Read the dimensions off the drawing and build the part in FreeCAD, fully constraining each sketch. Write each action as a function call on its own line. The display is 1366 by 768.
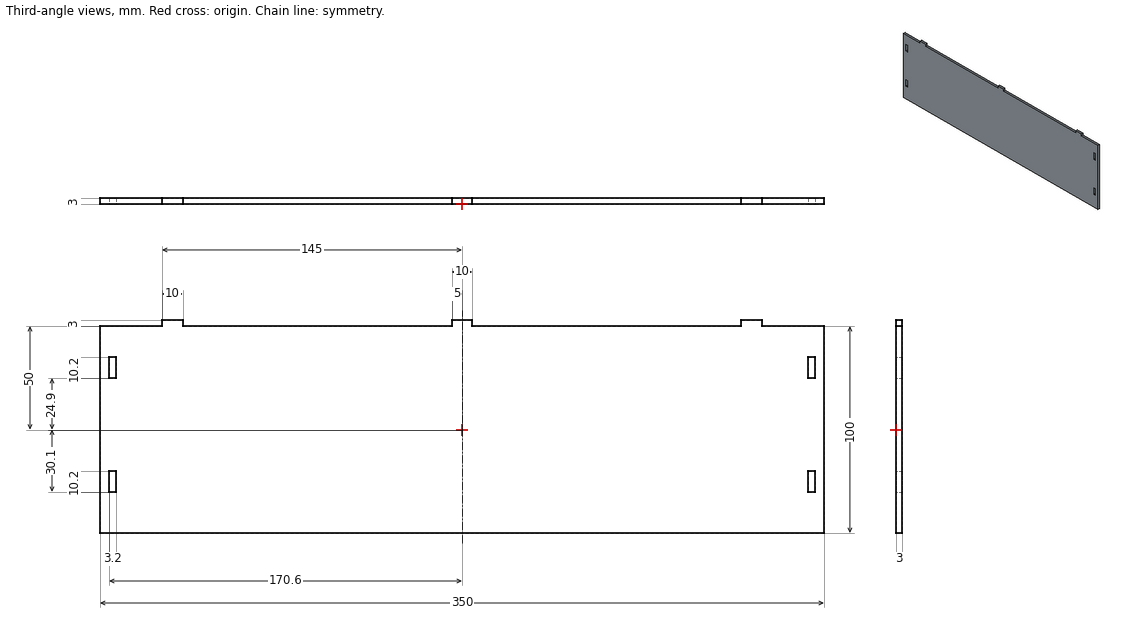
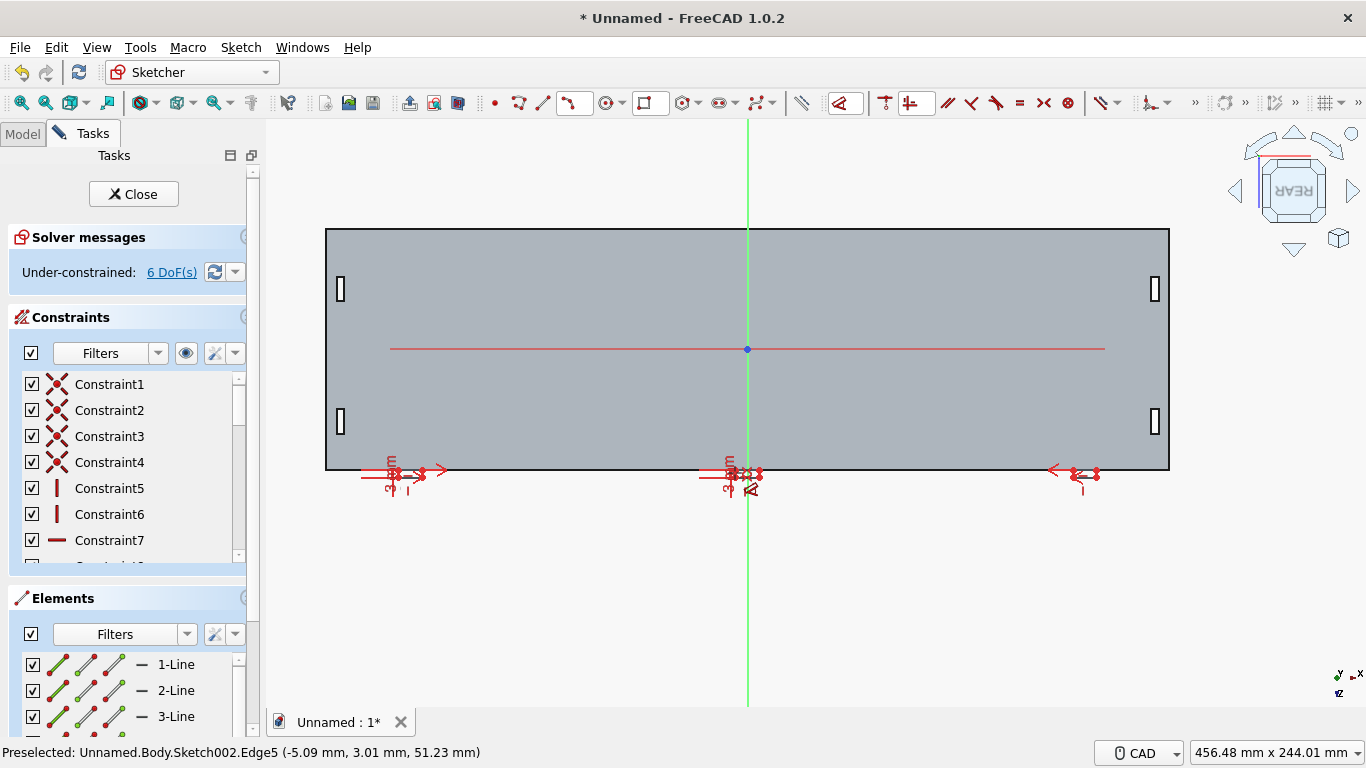
scroll(405, 478, up, 4)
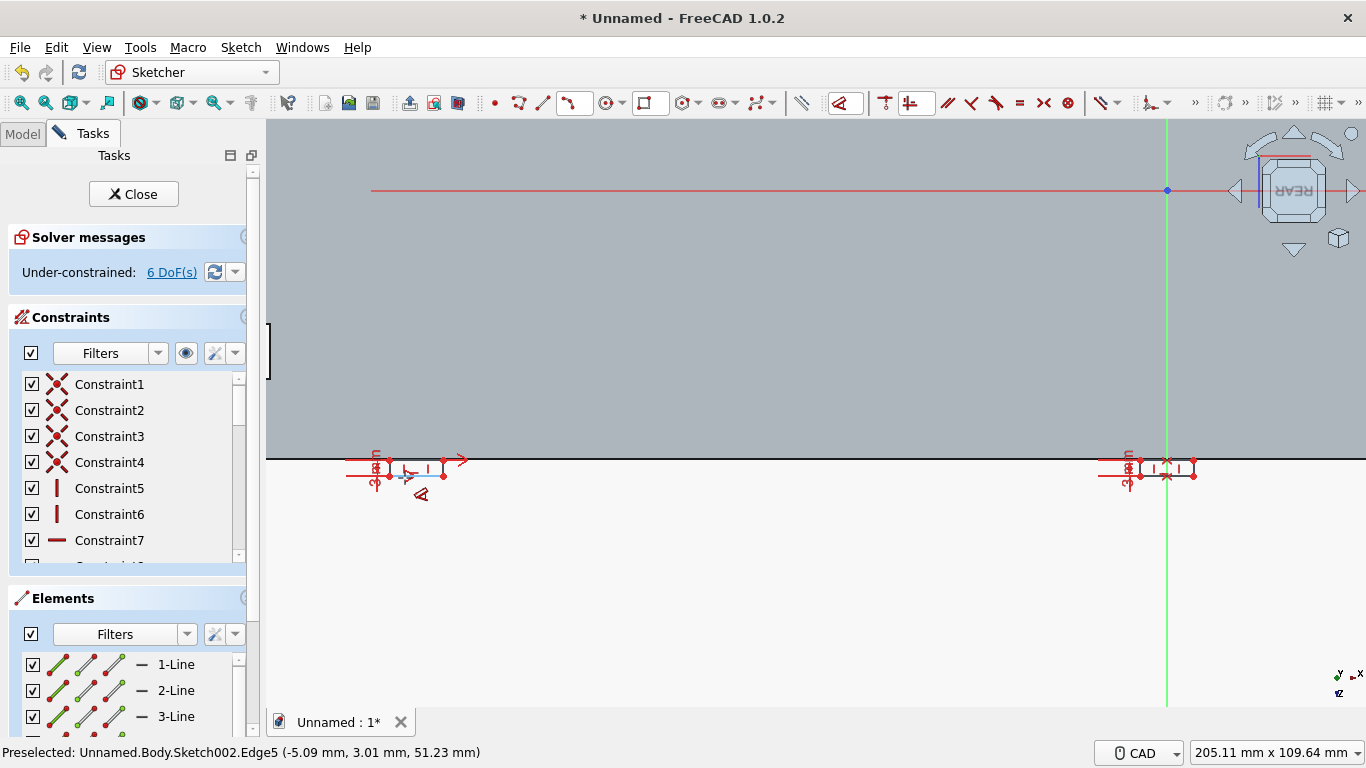
click(406, 476)
click(417, 510)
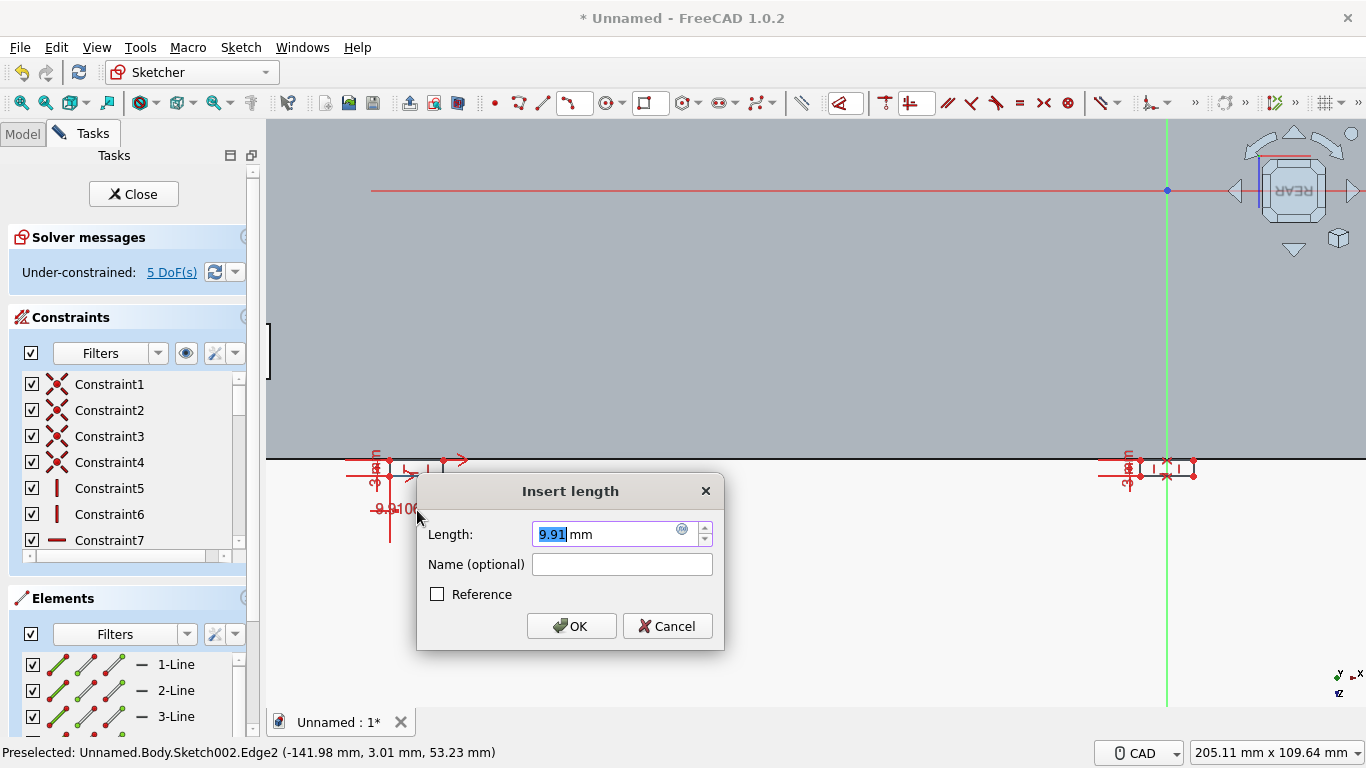
text(10)
key(Return)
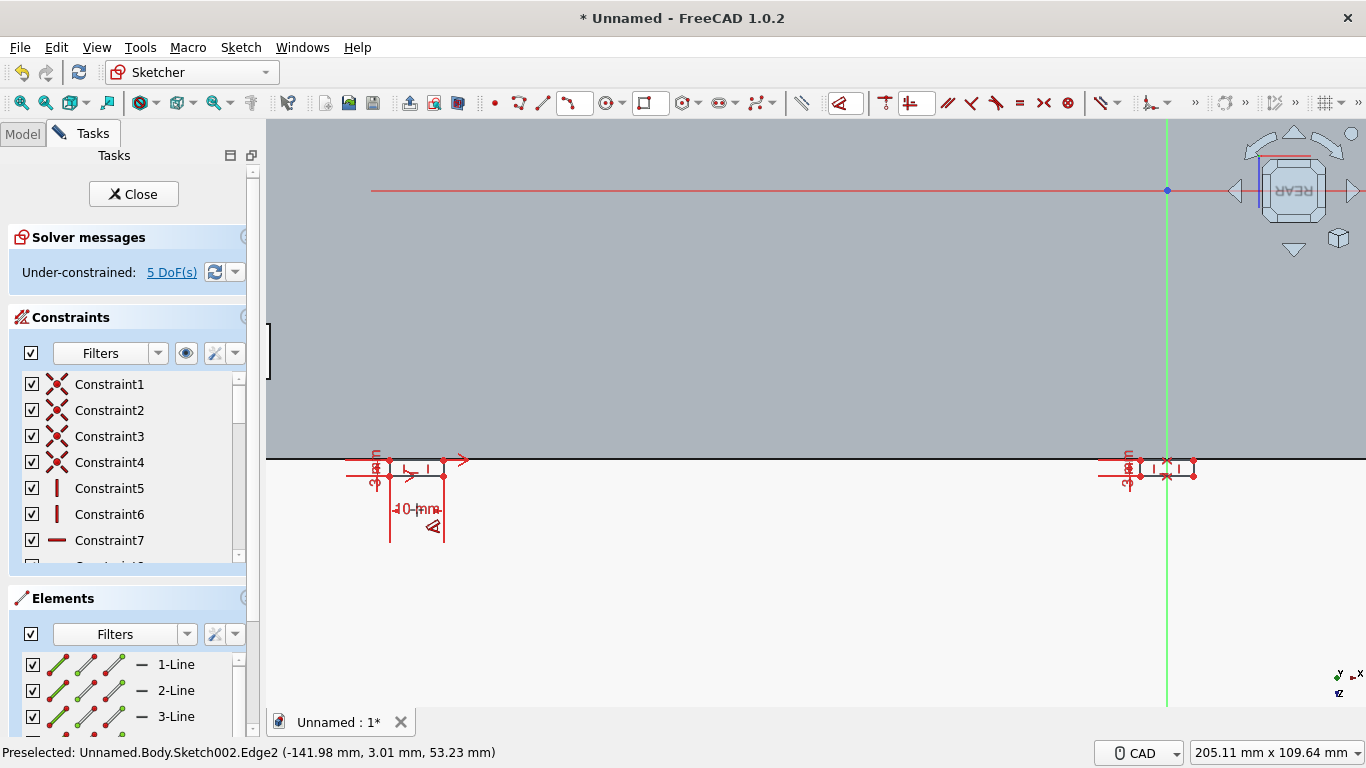
scroll(1156, 476, up, 2)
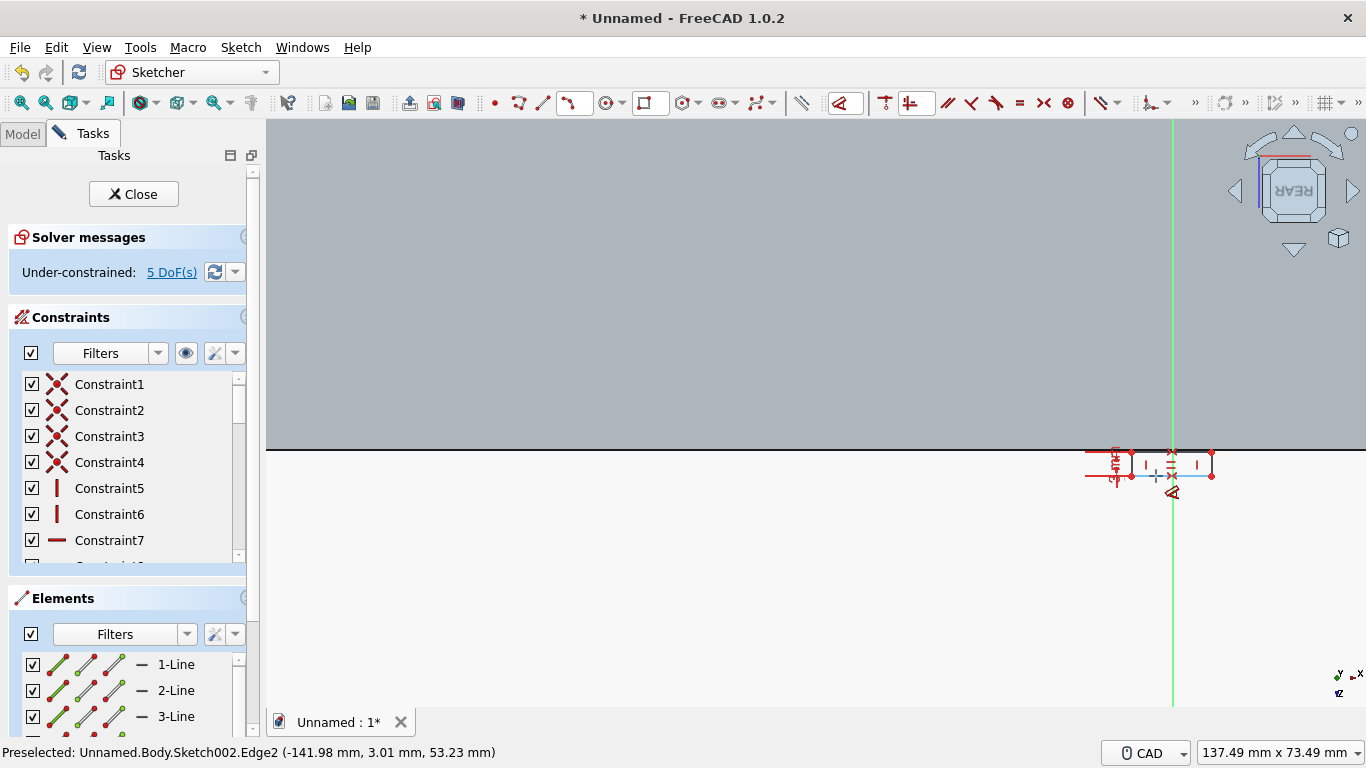
click(1156, 476)
click(1151, 510)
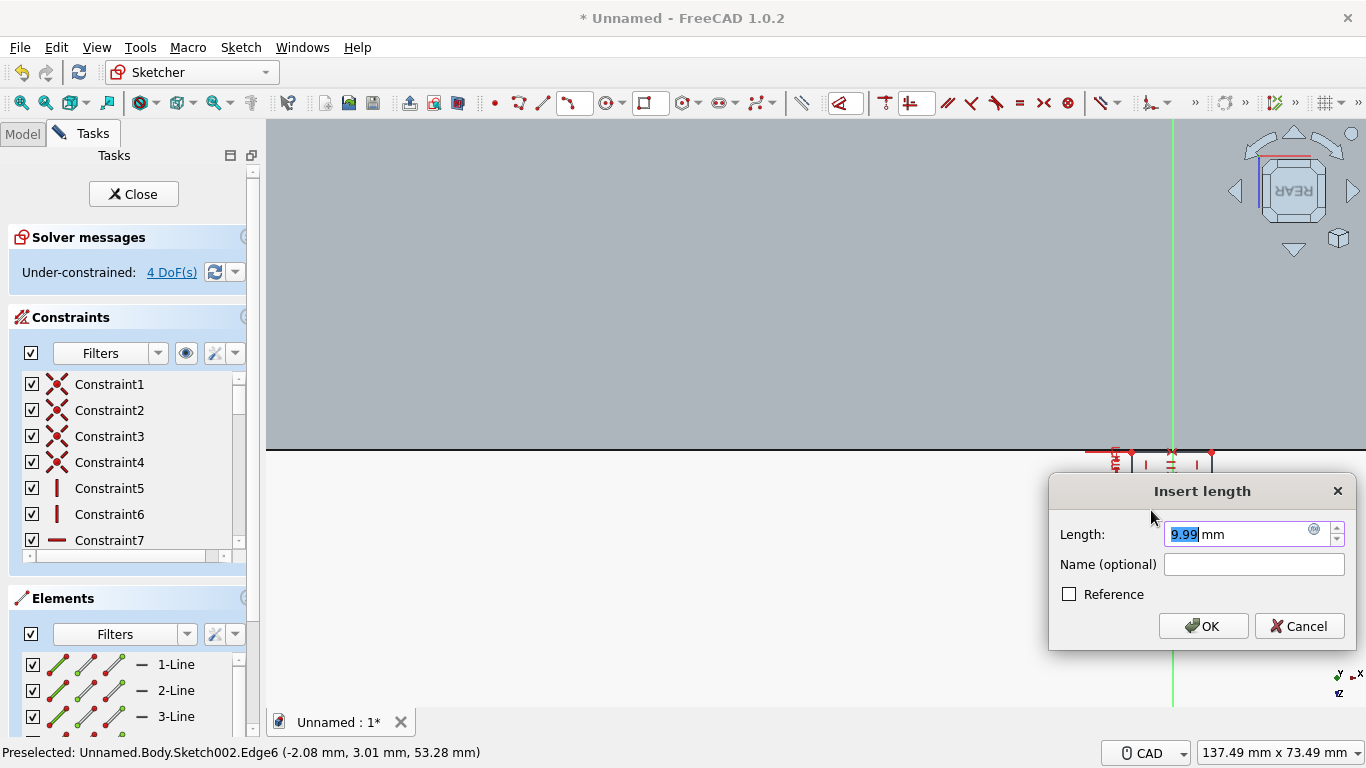
text(10)
key(Return)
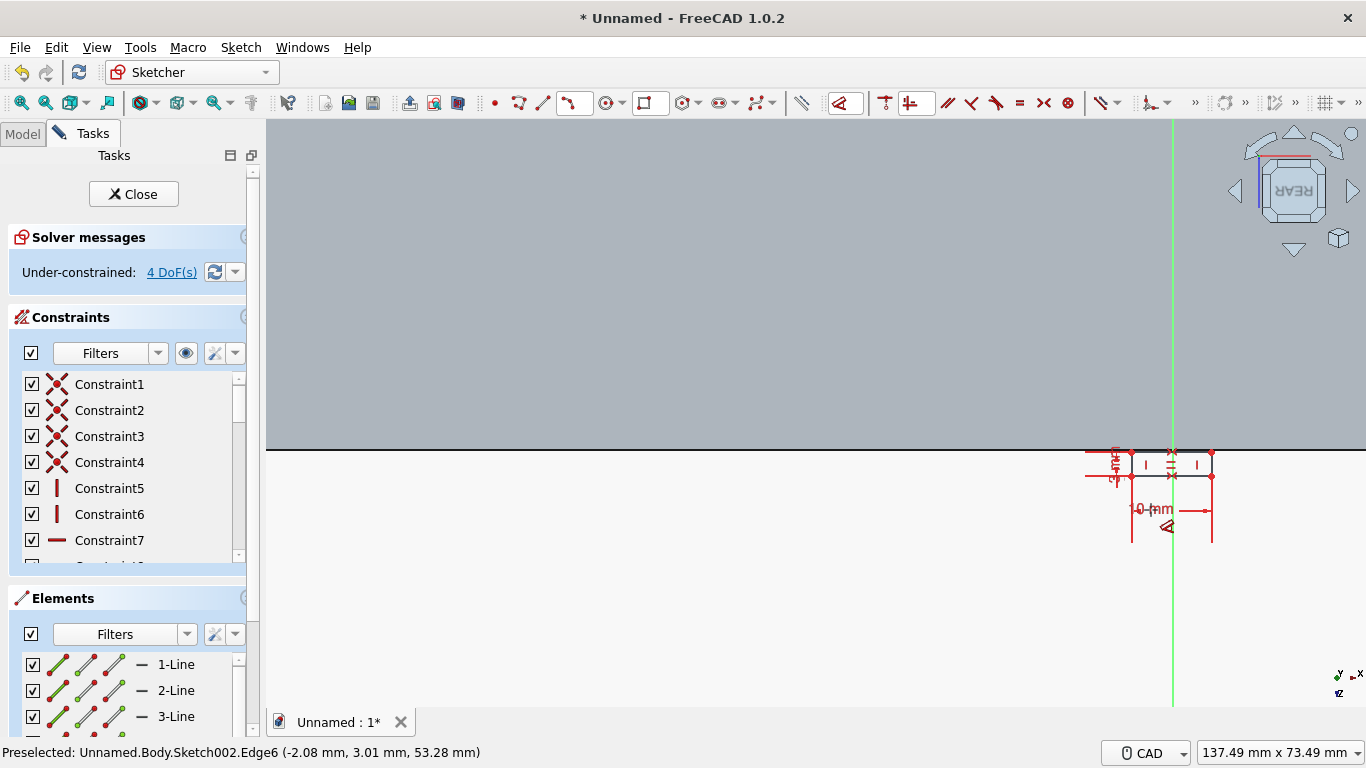
click(1132, 452)
click(1152, 534)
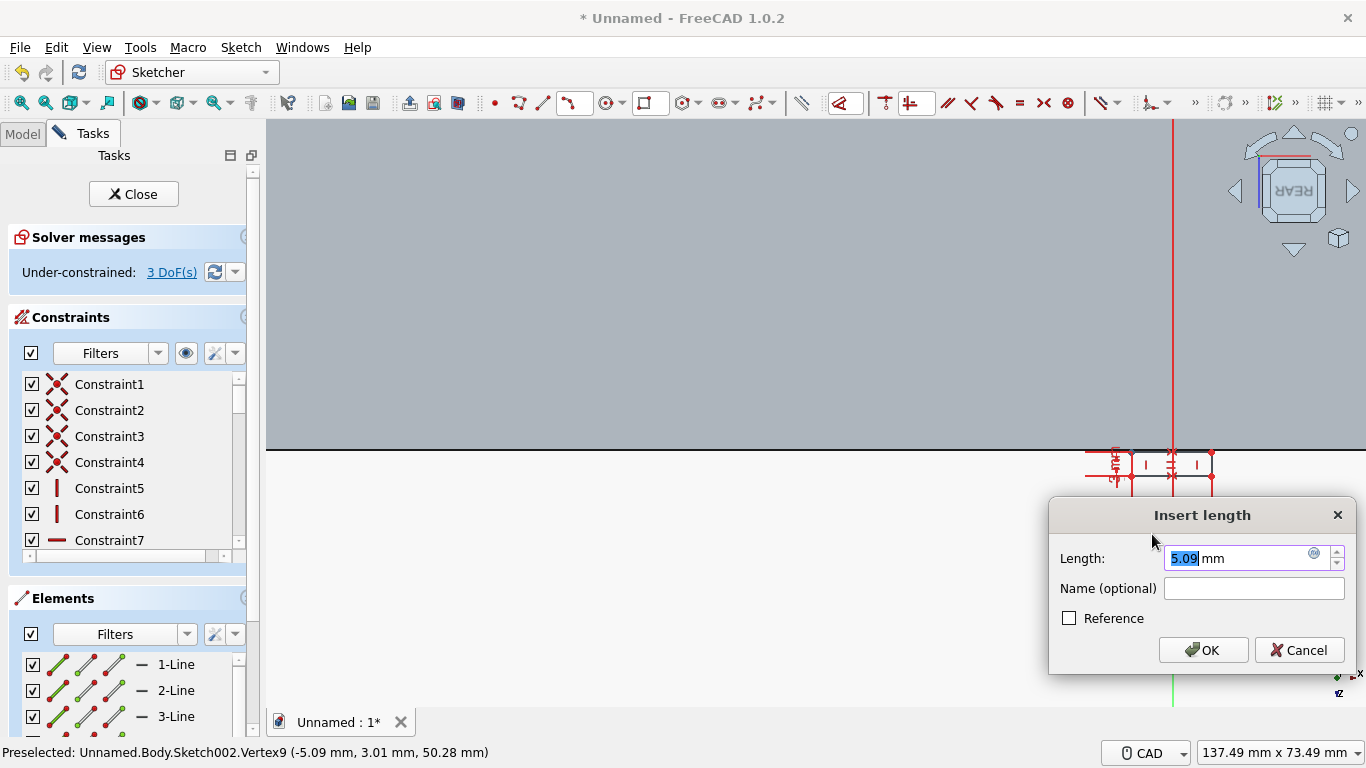
text(5)
key(Return)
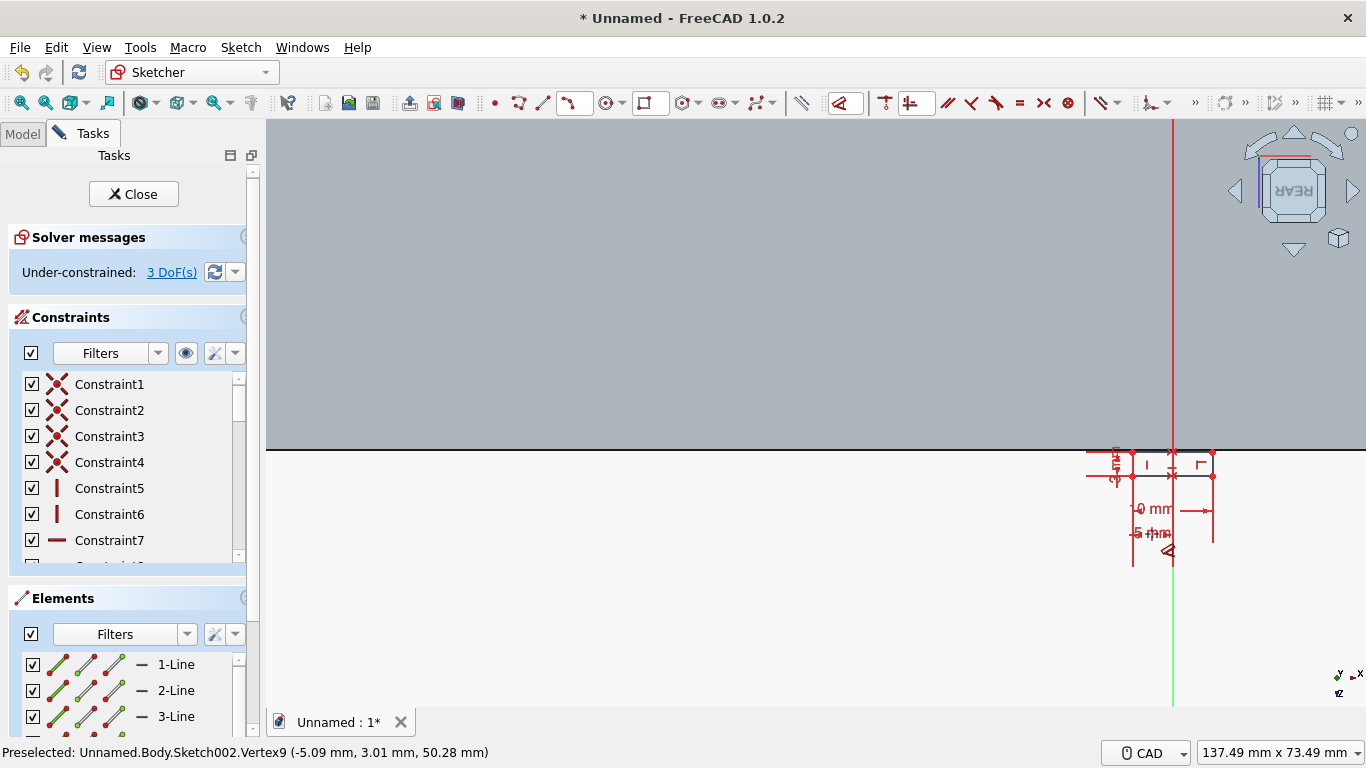
scroll(564, 478, down, 6)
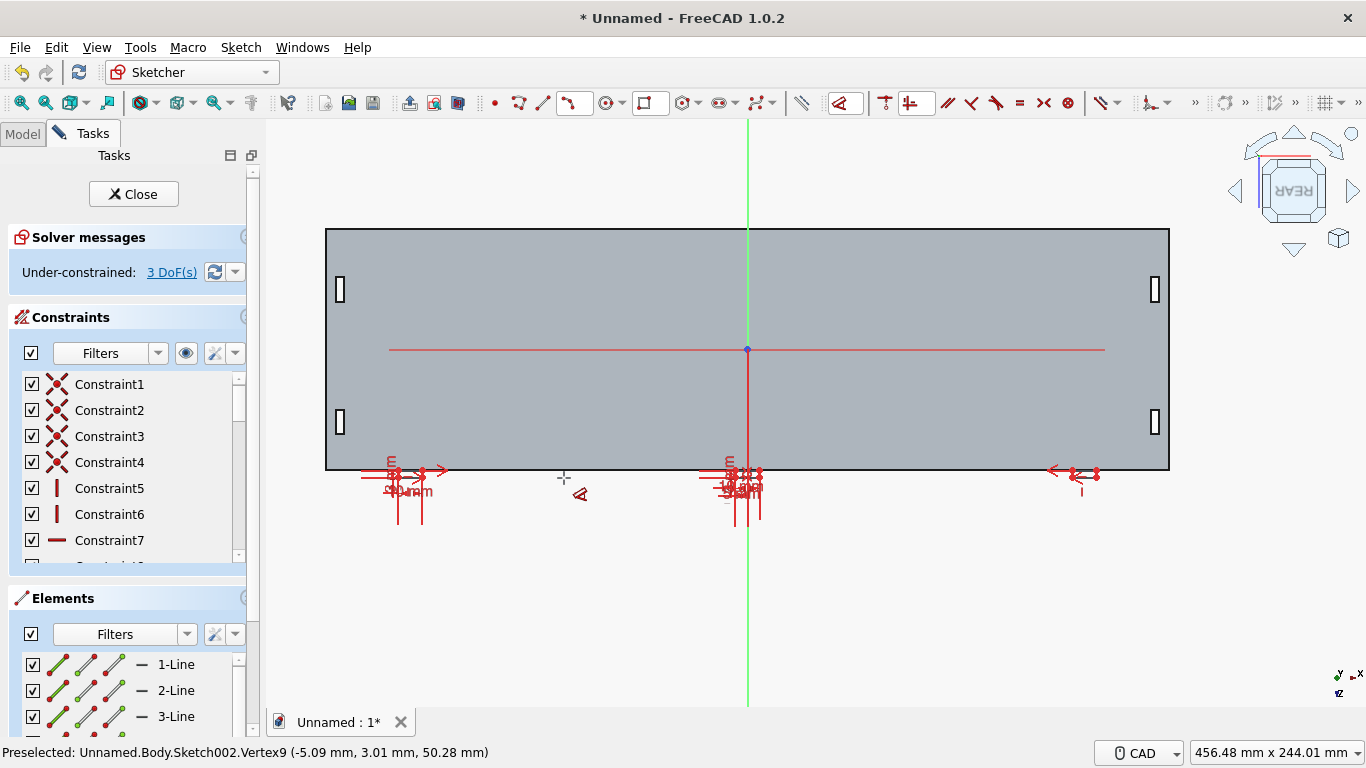
scroll(398, 471, up, 3)